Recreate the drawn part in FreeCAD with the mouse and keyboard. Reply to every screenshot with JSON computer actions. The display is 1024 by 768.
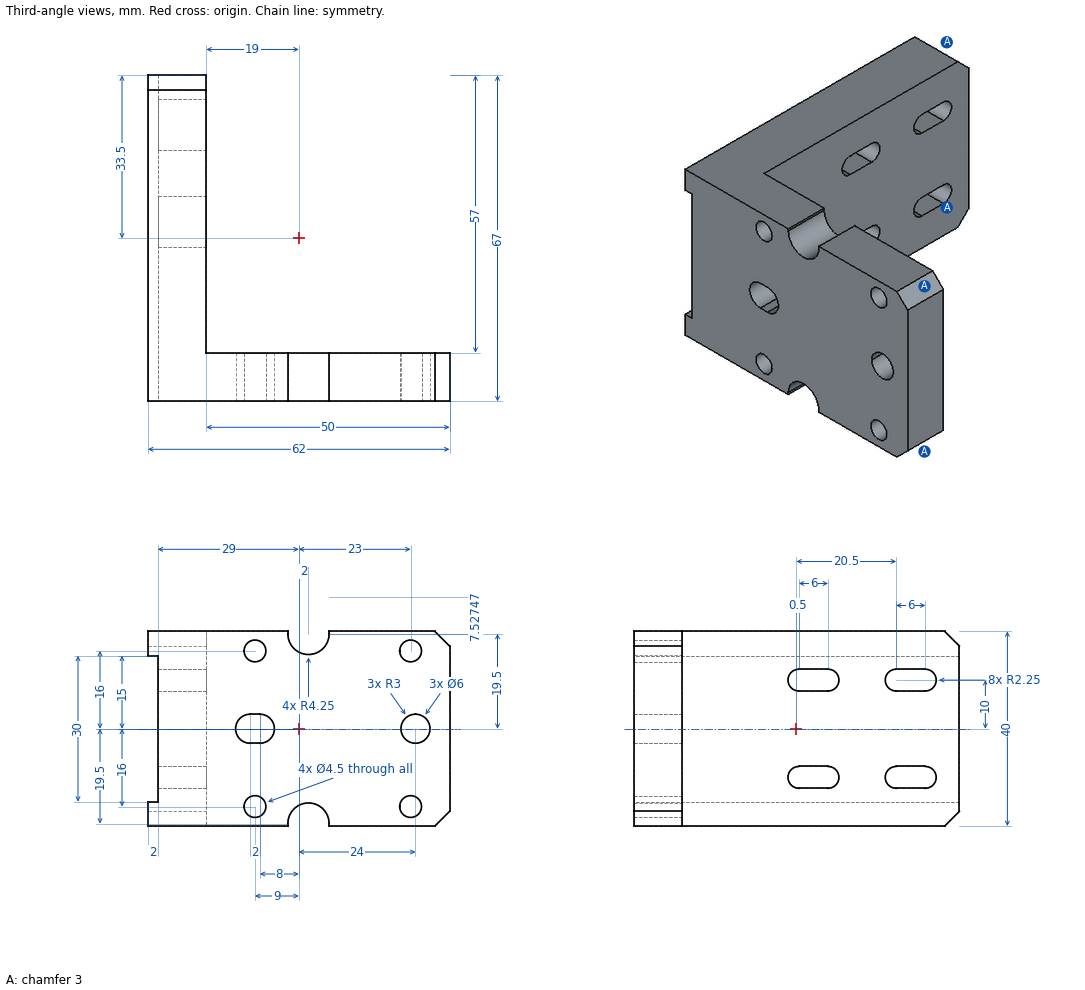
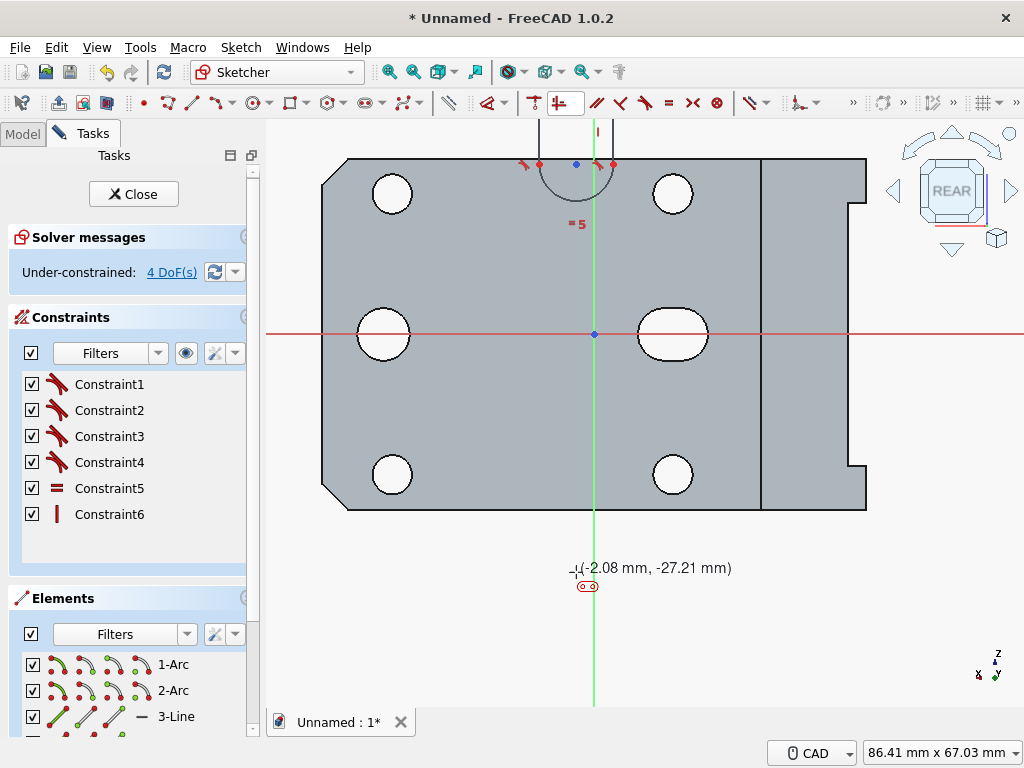
{"action": "left_click", "coordinate": [576, 572]}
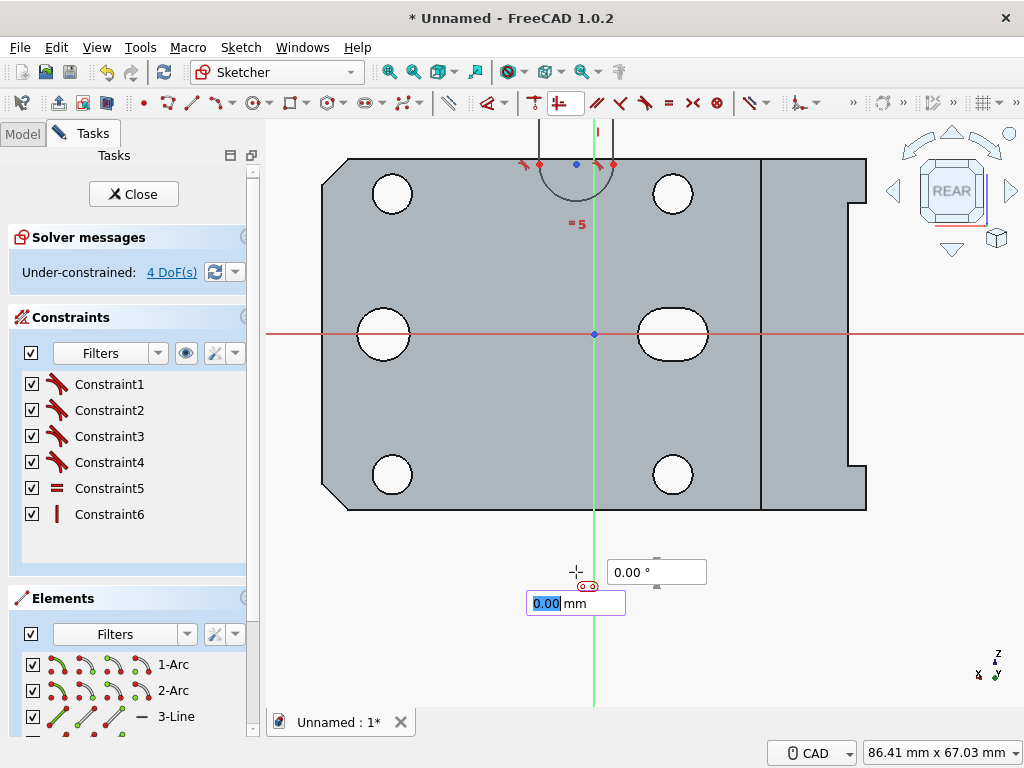
{"action": "left_click", "coordinate": [576, 505]}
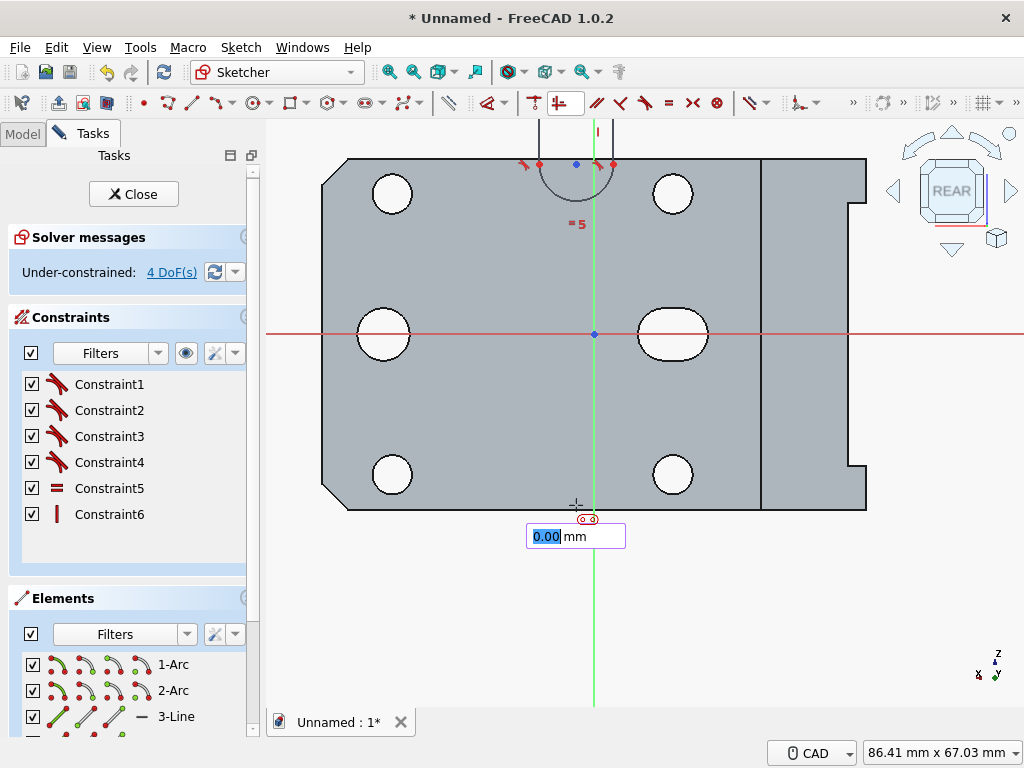
{"action": "left_click", "coordinate": [614, 538]}
{"action": "key", "text": "Escape"}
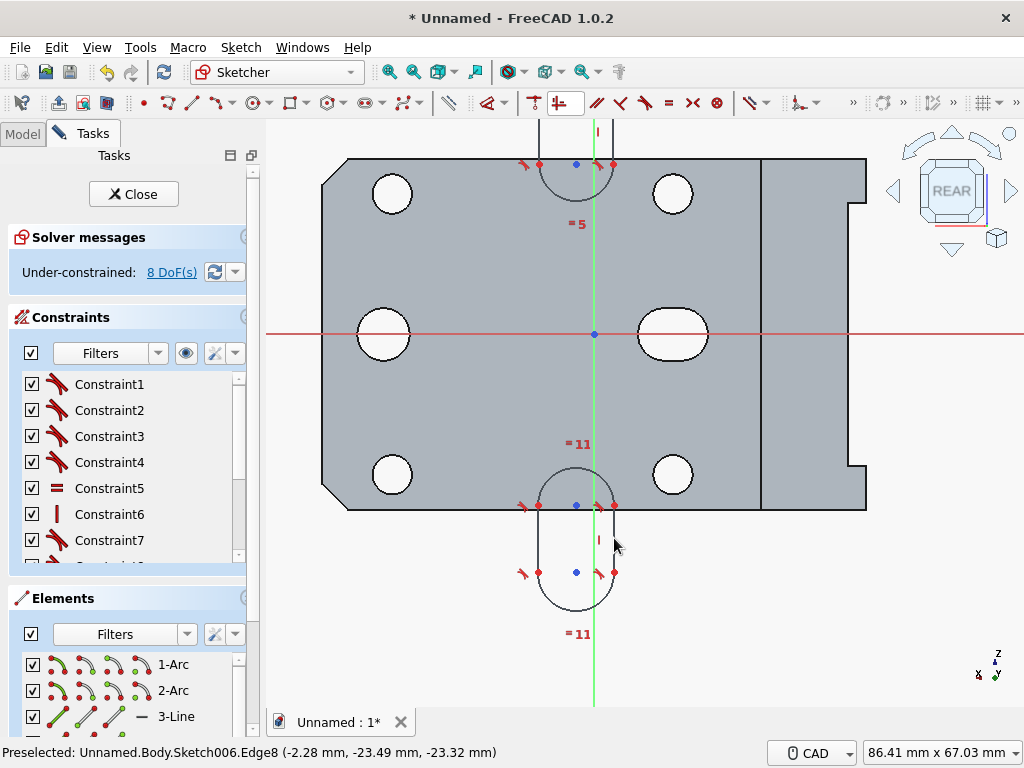
{"action": "left_click", "coordinate": [555, 194]}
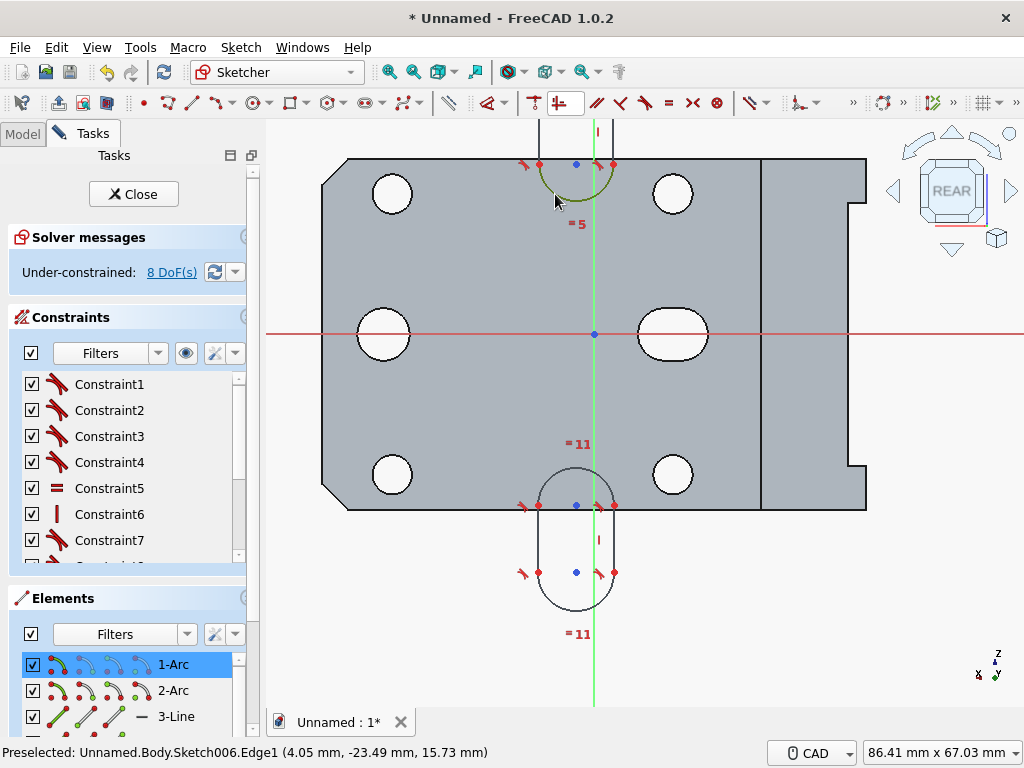
{"action": "left_click", "coordinate": [554, 604]}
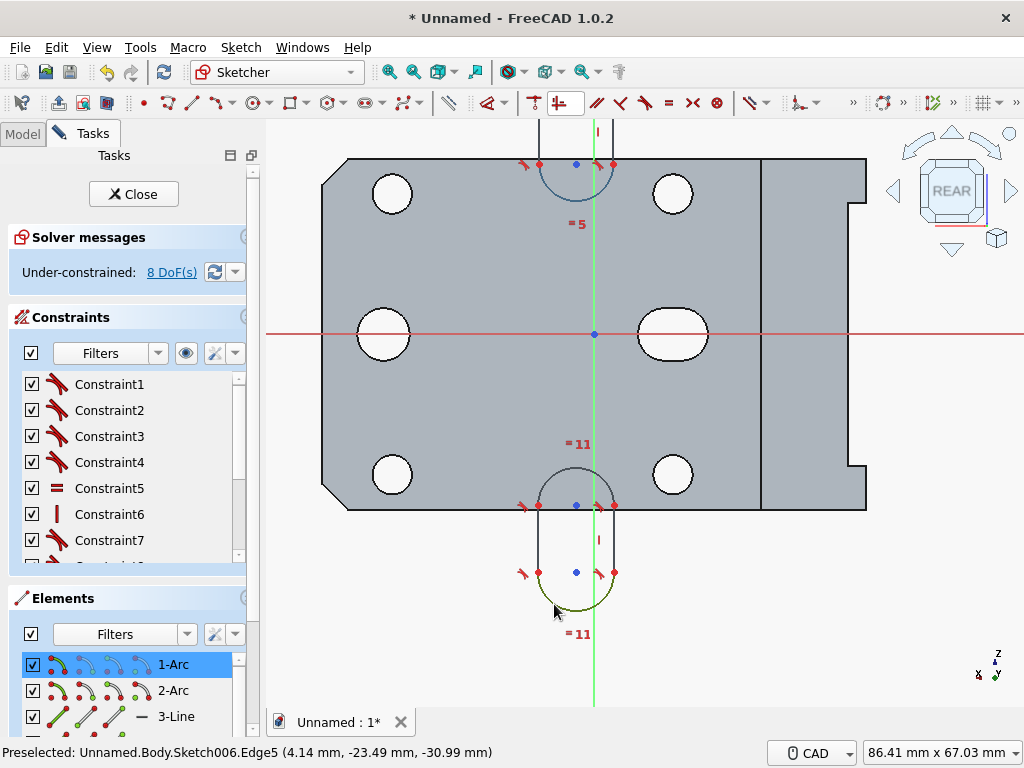
{"action": "left_click", "coordinate": [670, 104]}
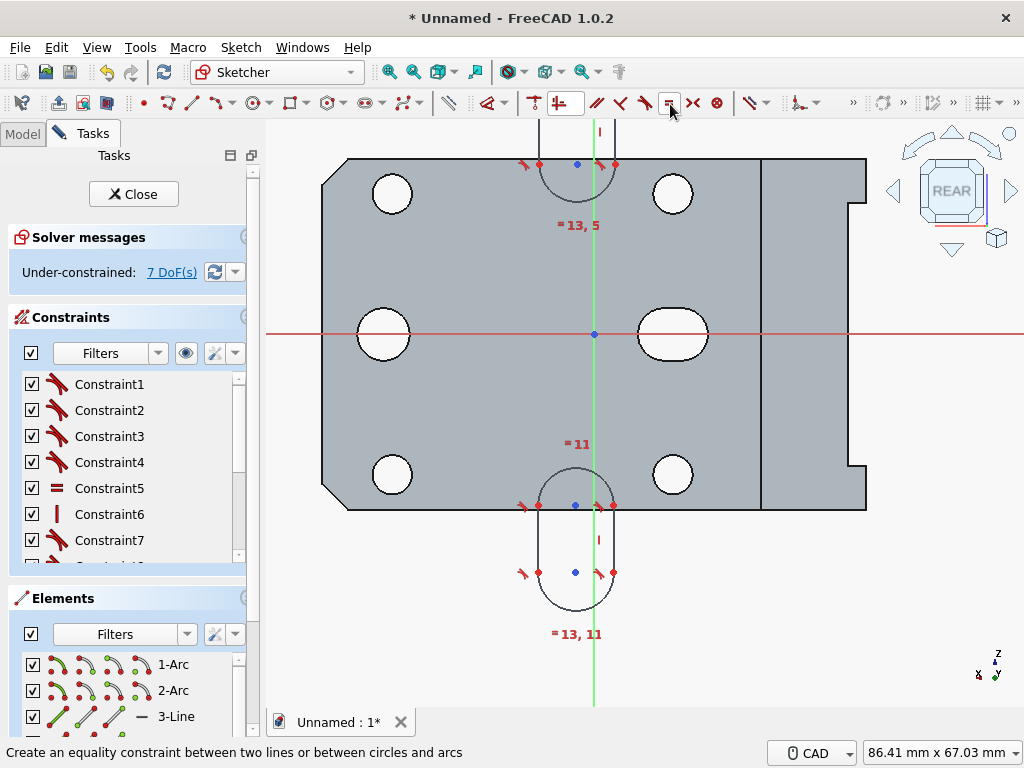
{"action": "scroll", "coordinate": [577, 573], "scroll_direction": "down", "scroll_amount": 2}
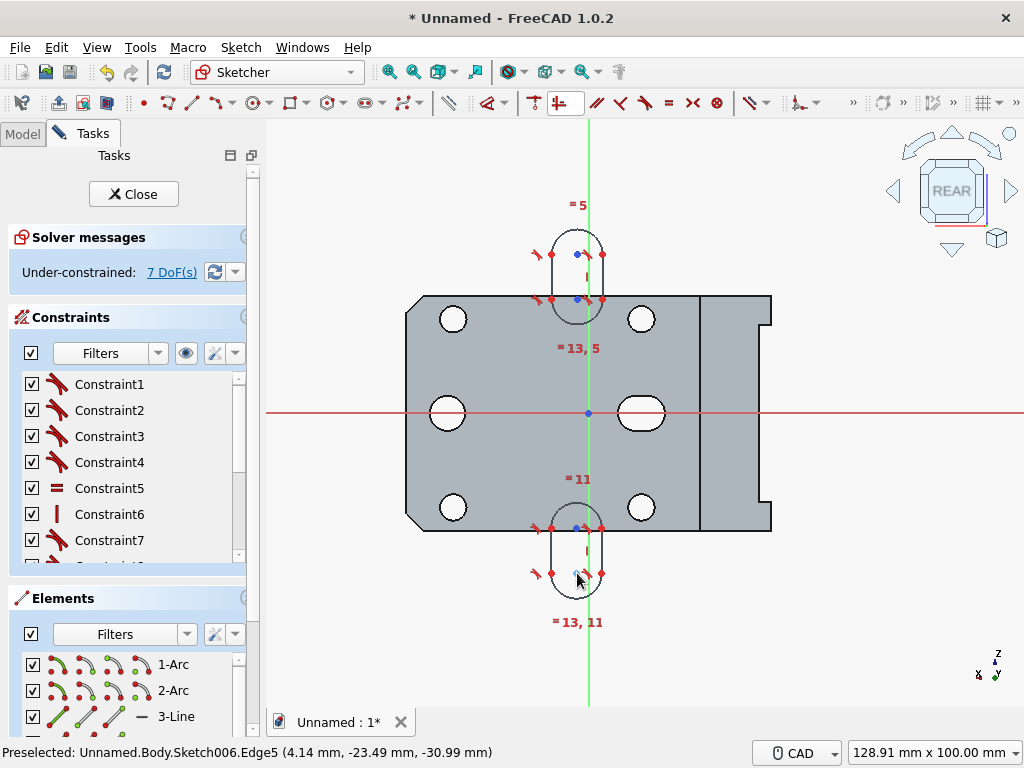
{"action": "left_click", "coordinate": [577, 255]}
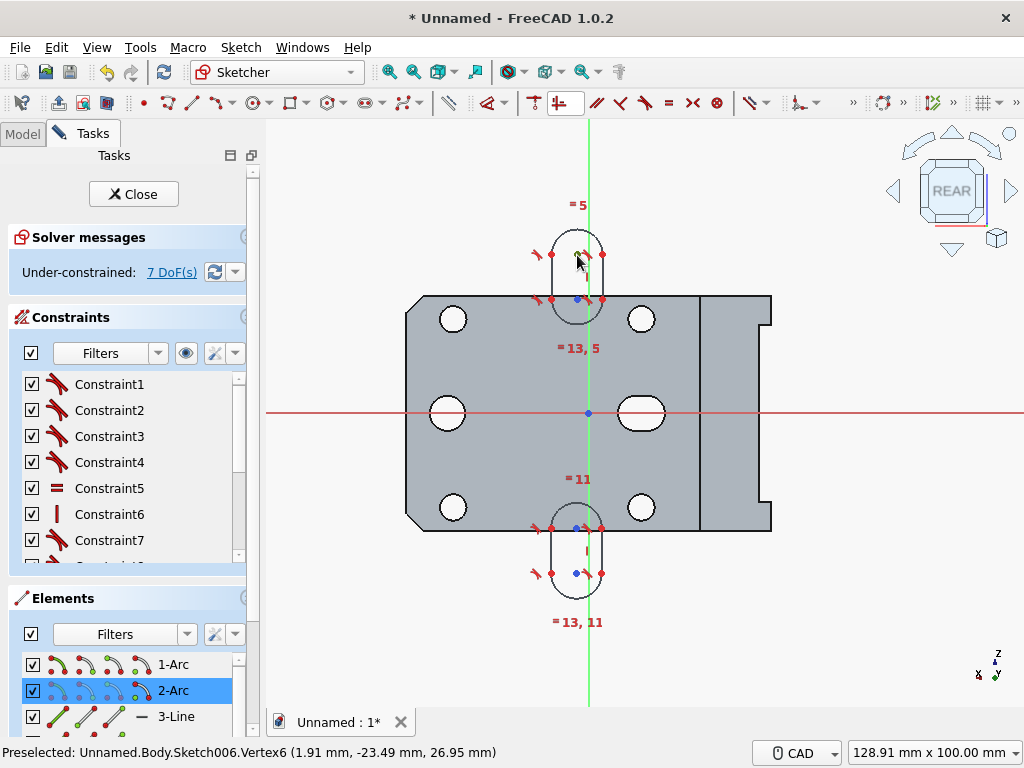
{"action": "left_click", "coordinate": [576, 573]}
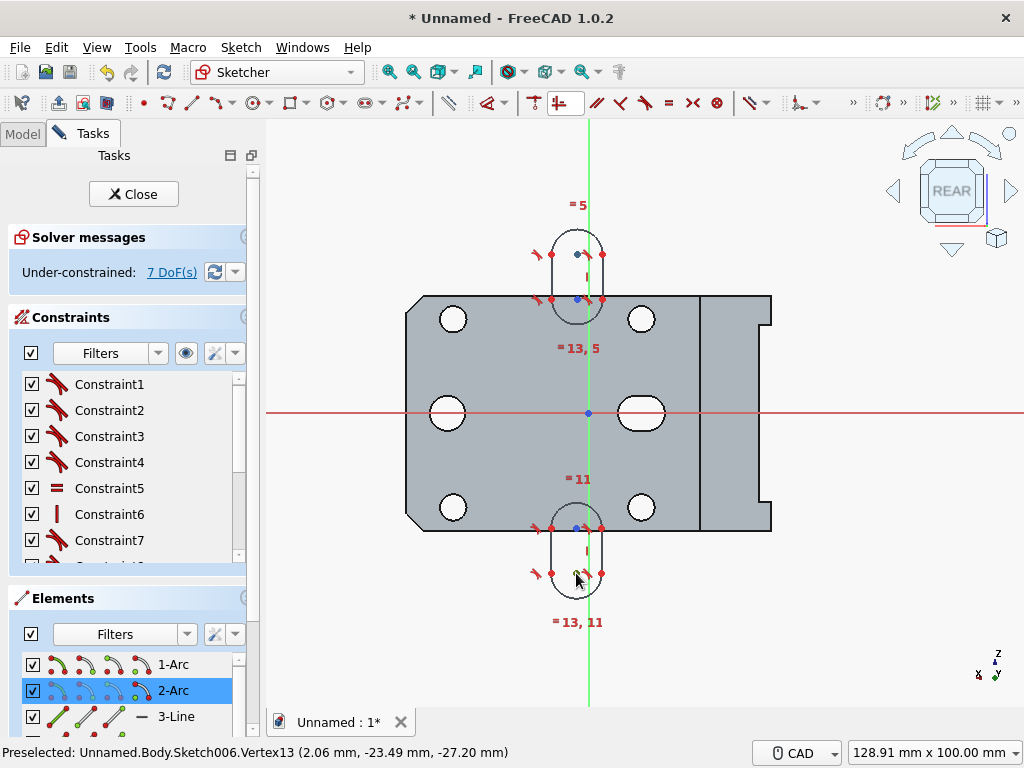
{"action": "left_click", "coordinate": [334, 413]}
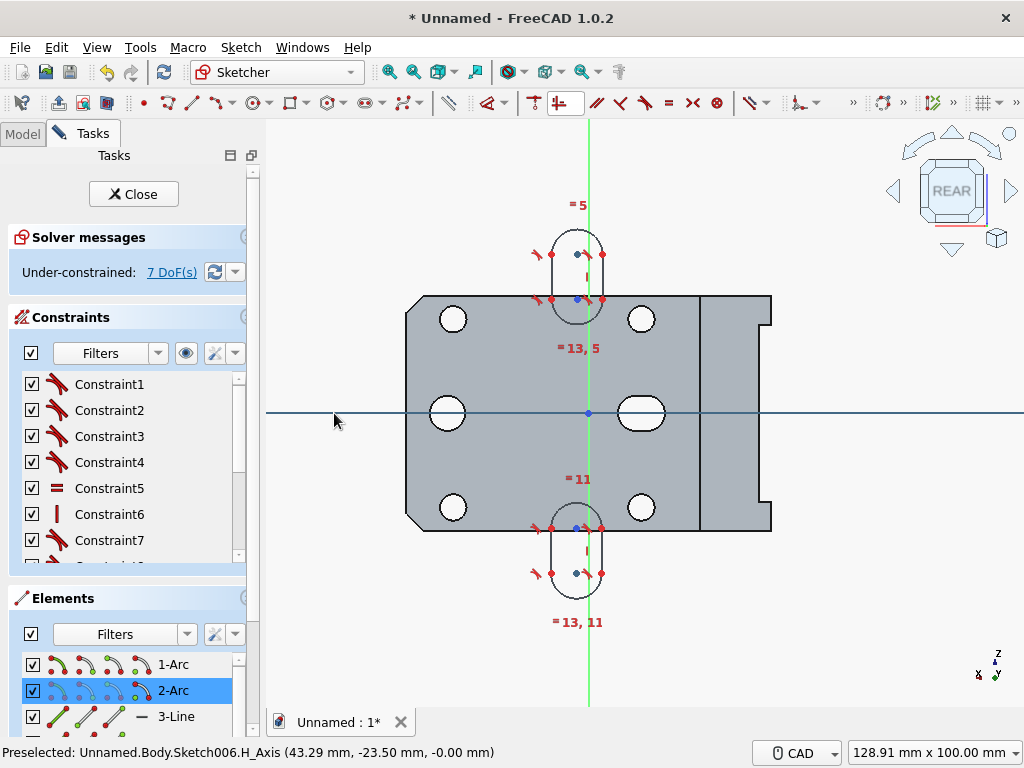
{"action": "left_click", "coordinate": [694, 104]}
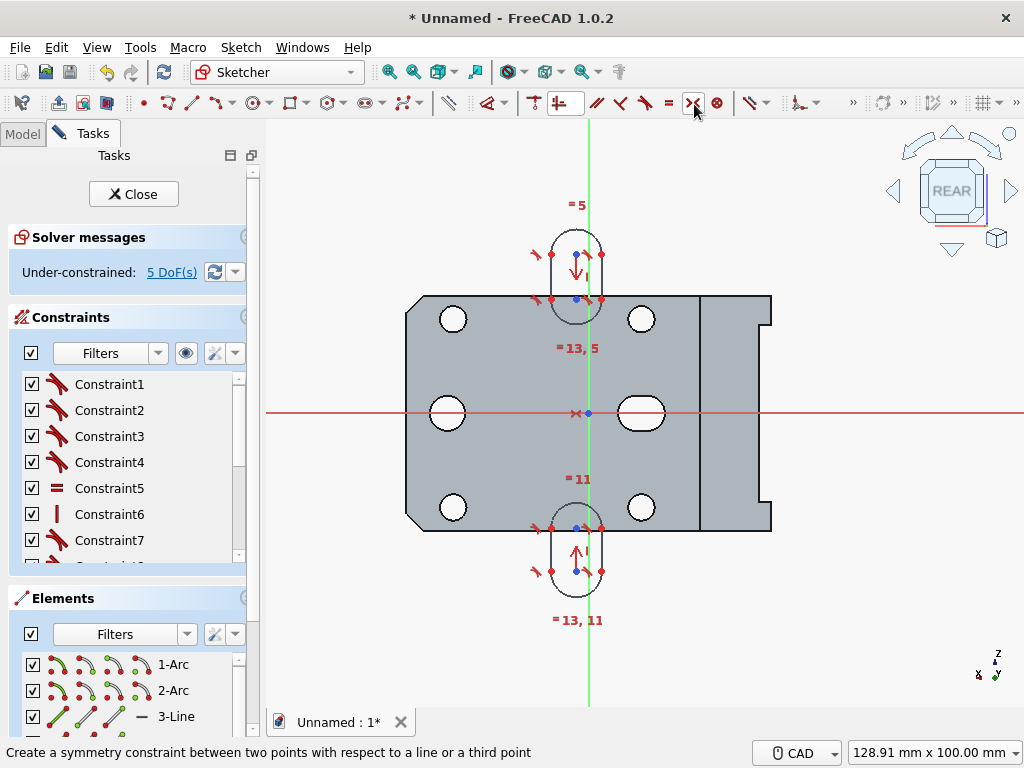
{"action": "left_click", "coordinate": [488, 104]}